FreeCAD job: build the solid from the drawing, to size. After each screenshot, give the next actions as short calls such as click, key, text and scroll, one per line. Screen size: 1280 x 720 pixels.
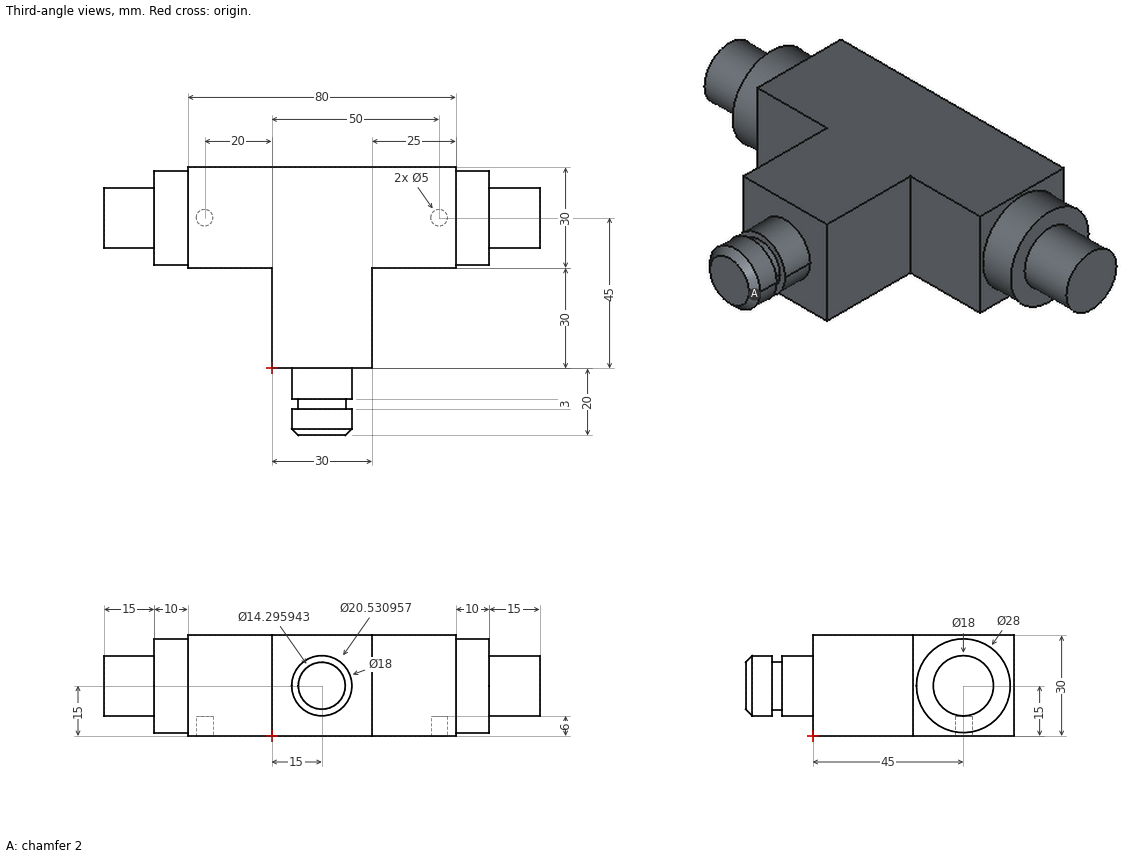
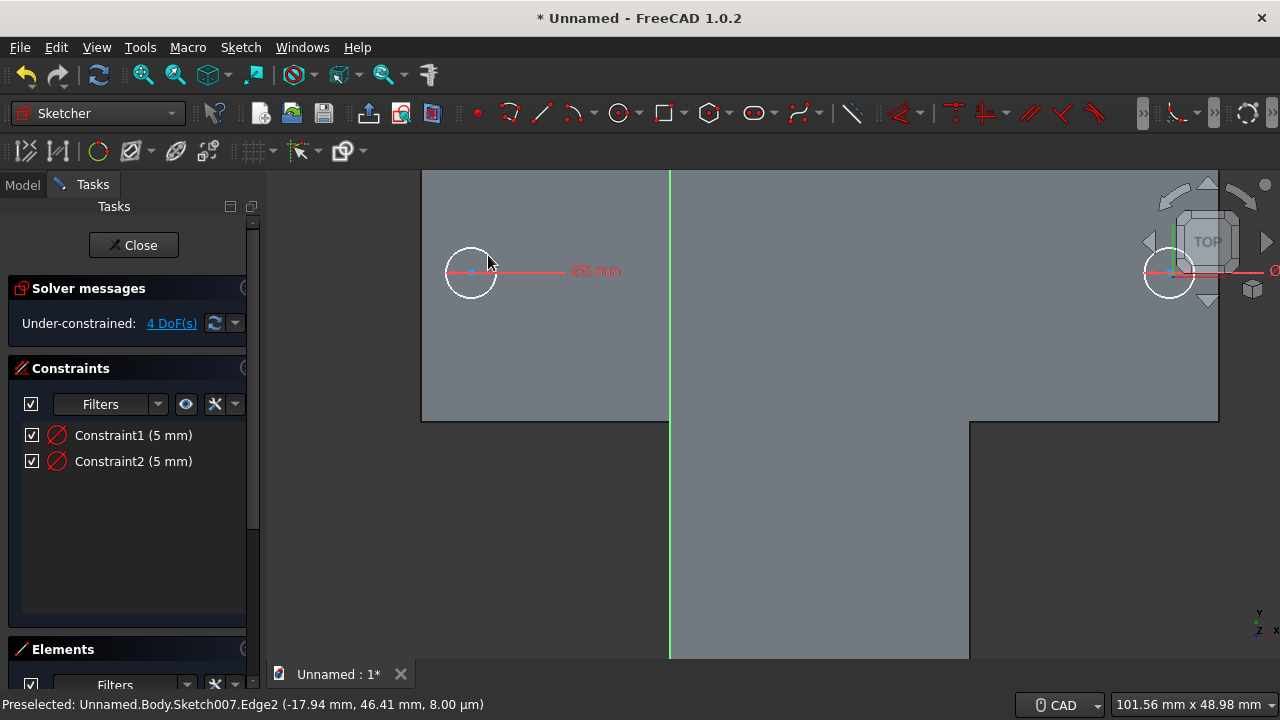
key(d)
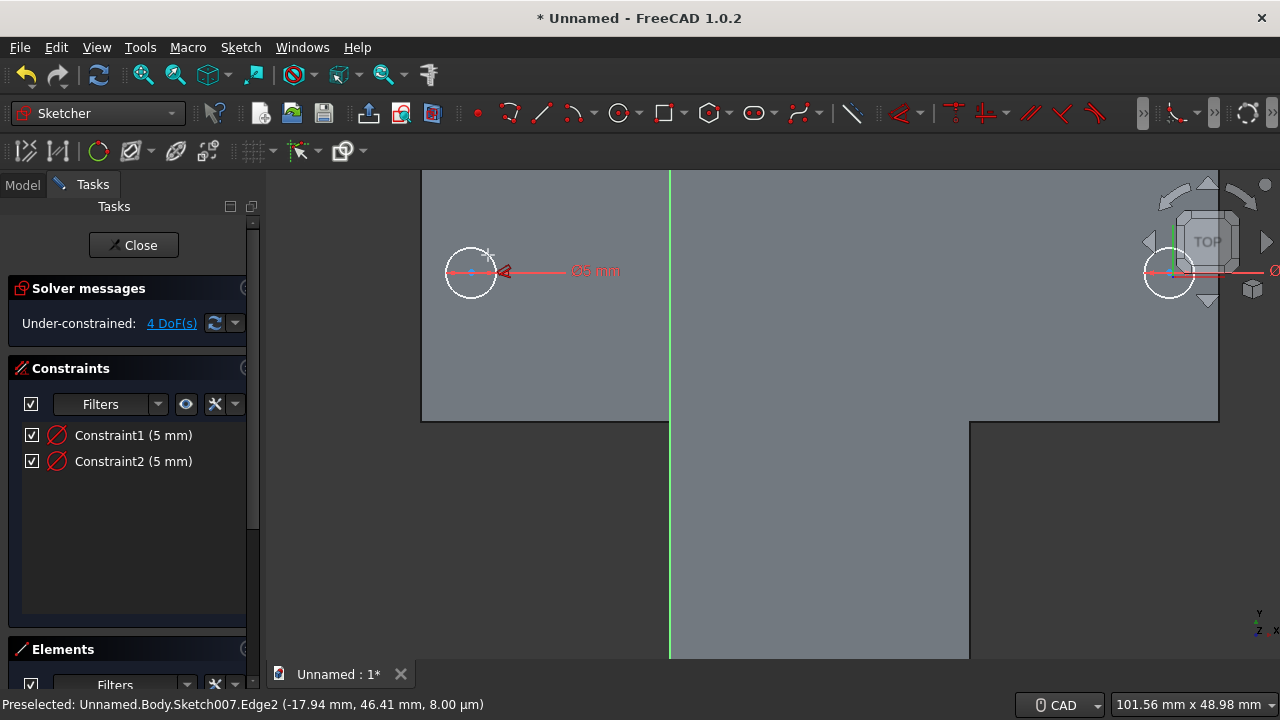
scroll(470, 272, down, 2)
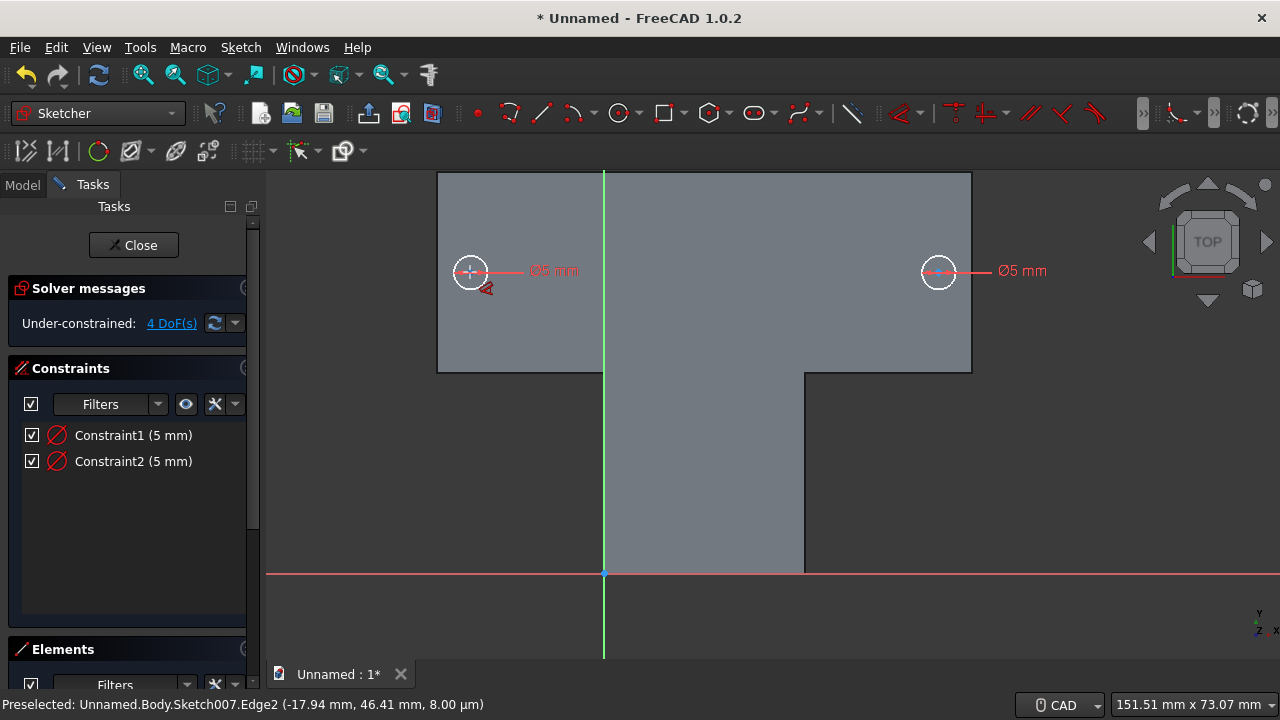
click(939, 273)
click(772, 608)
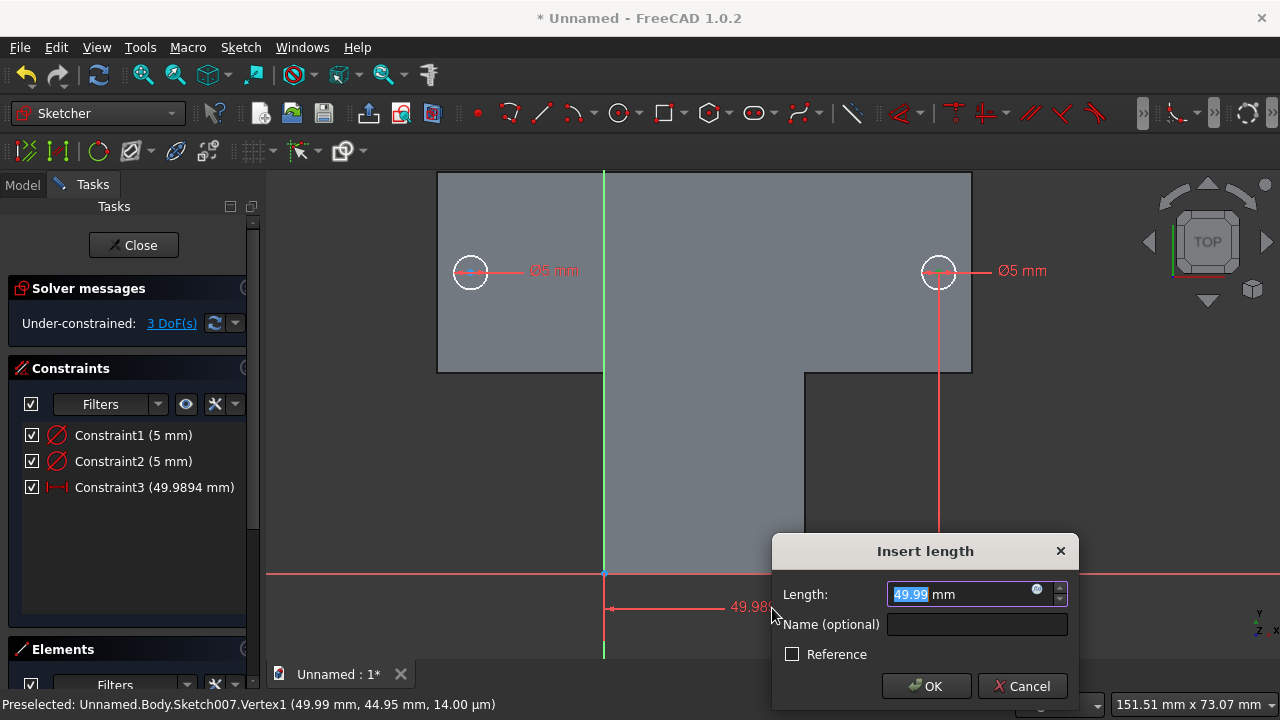
text(50)
key(Return)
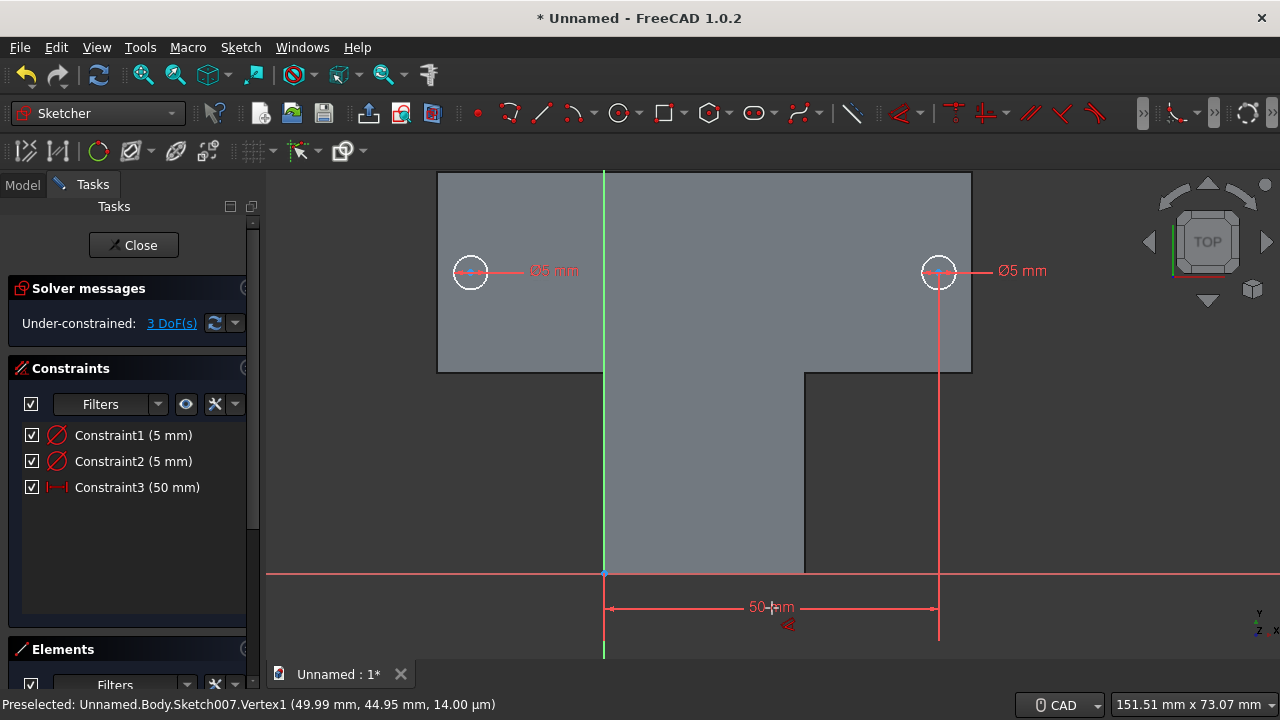
click(939, 273)
click(973, 423)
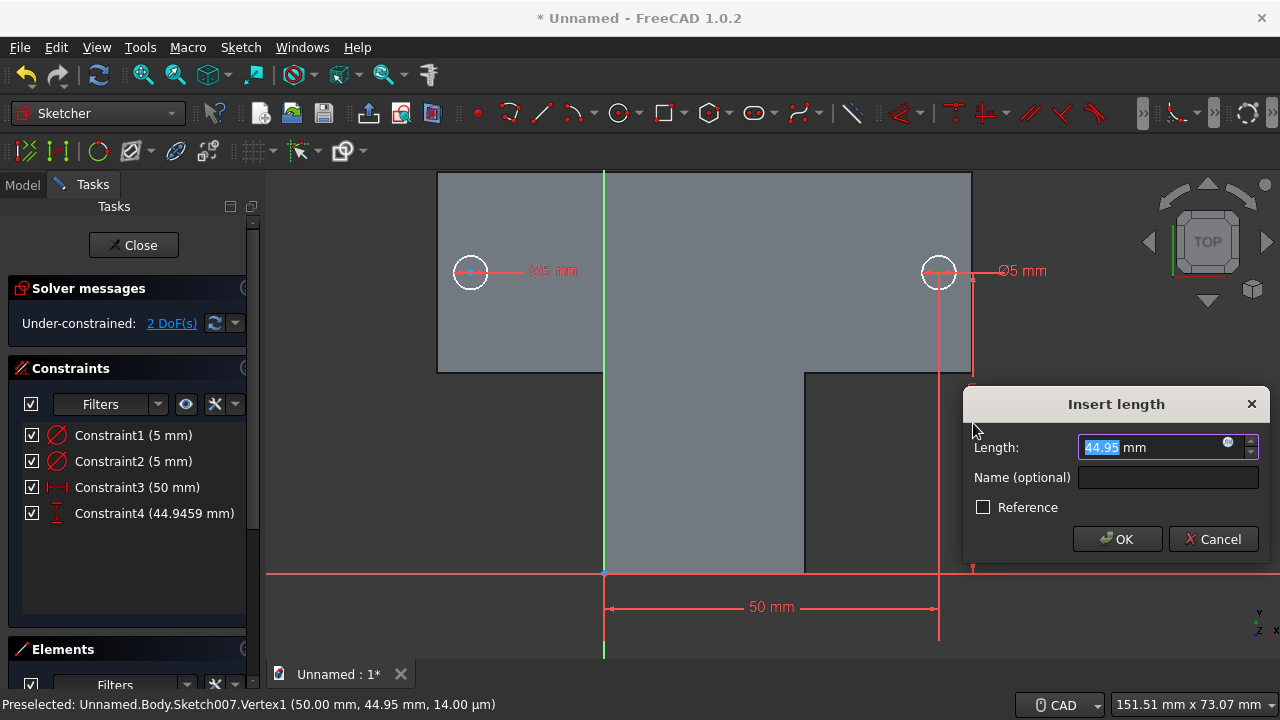
text(45)
key(Return)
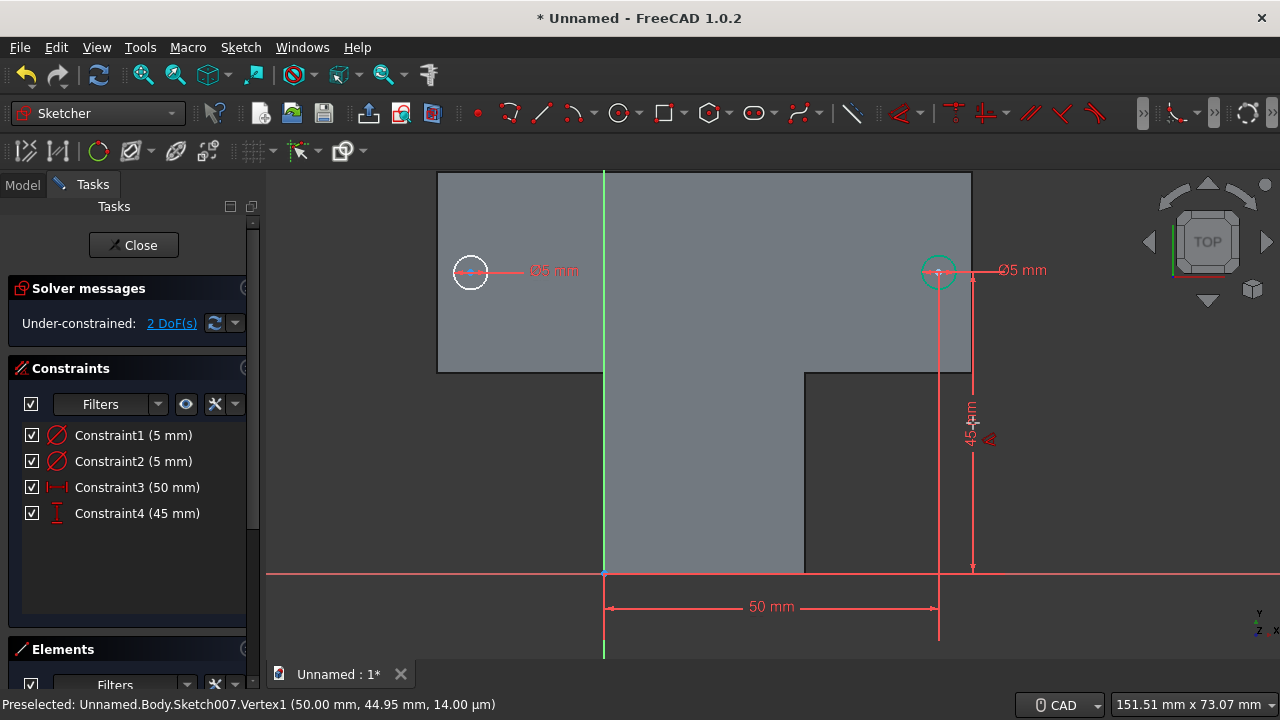
click(471, 273)
click(538, 608)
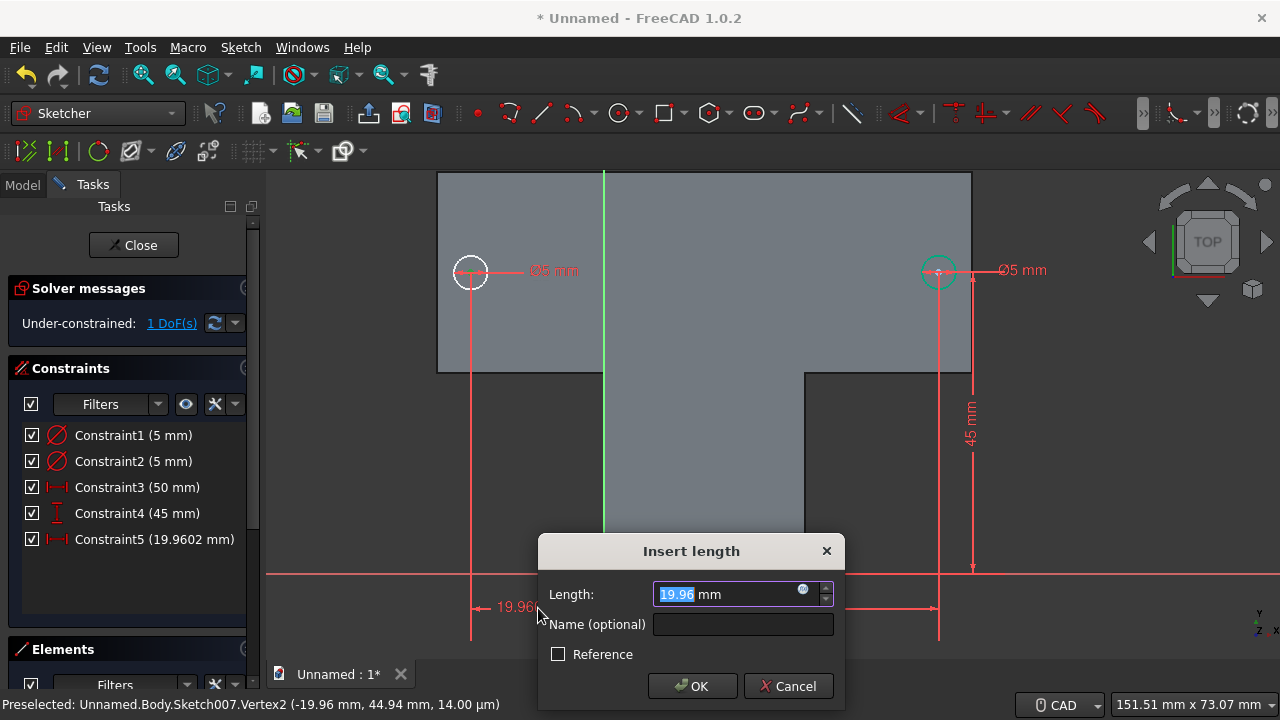
text(20)
key(Return)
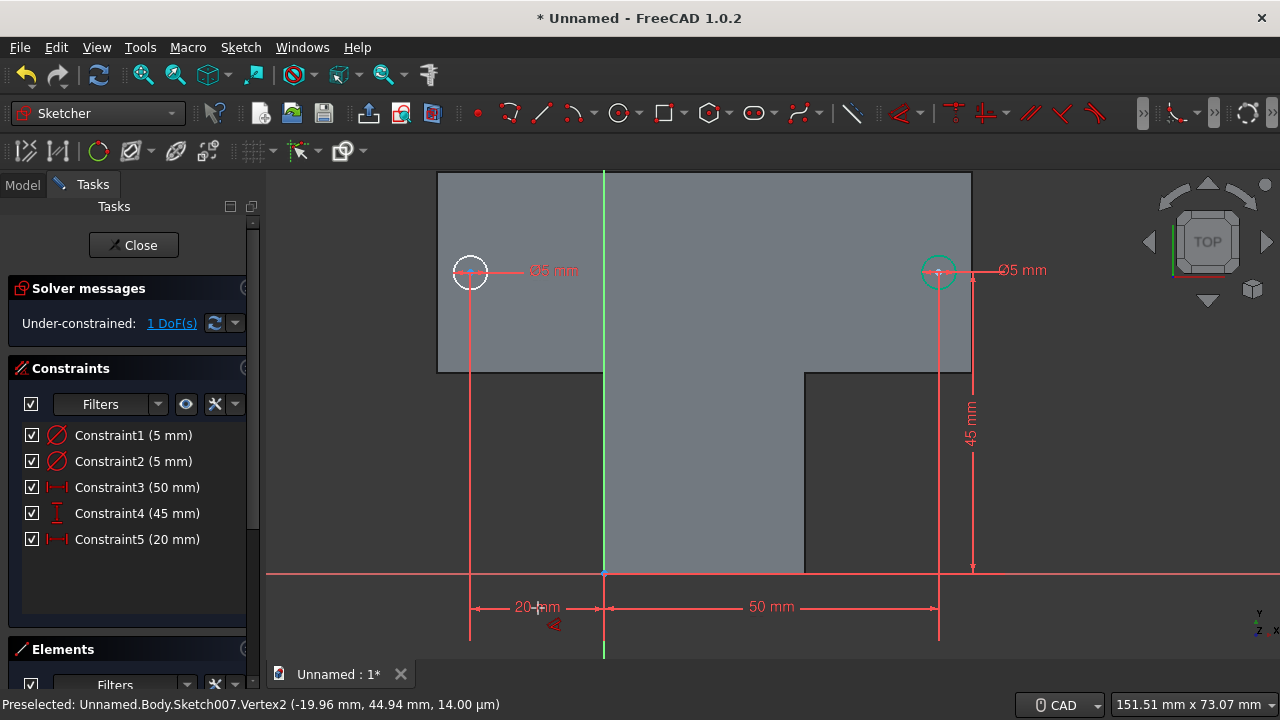
click(470, 273)
click(436, 423)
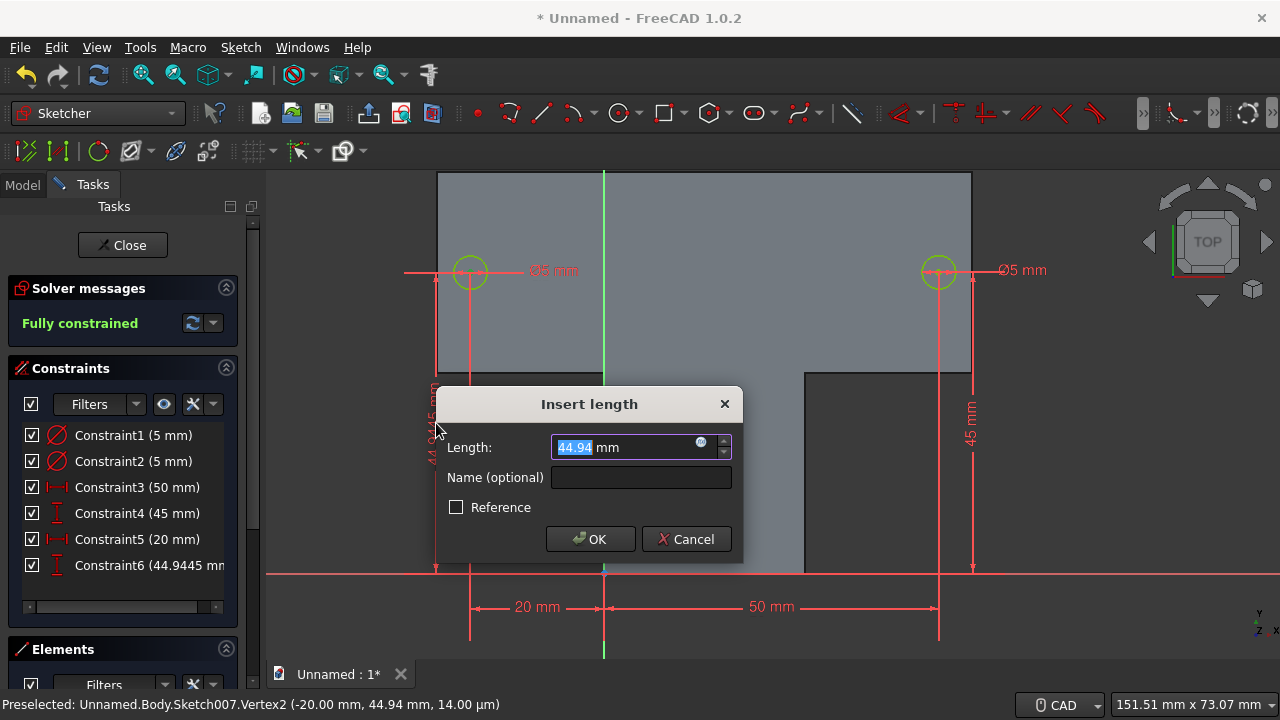
text(45)
key(Return)
key(Escape)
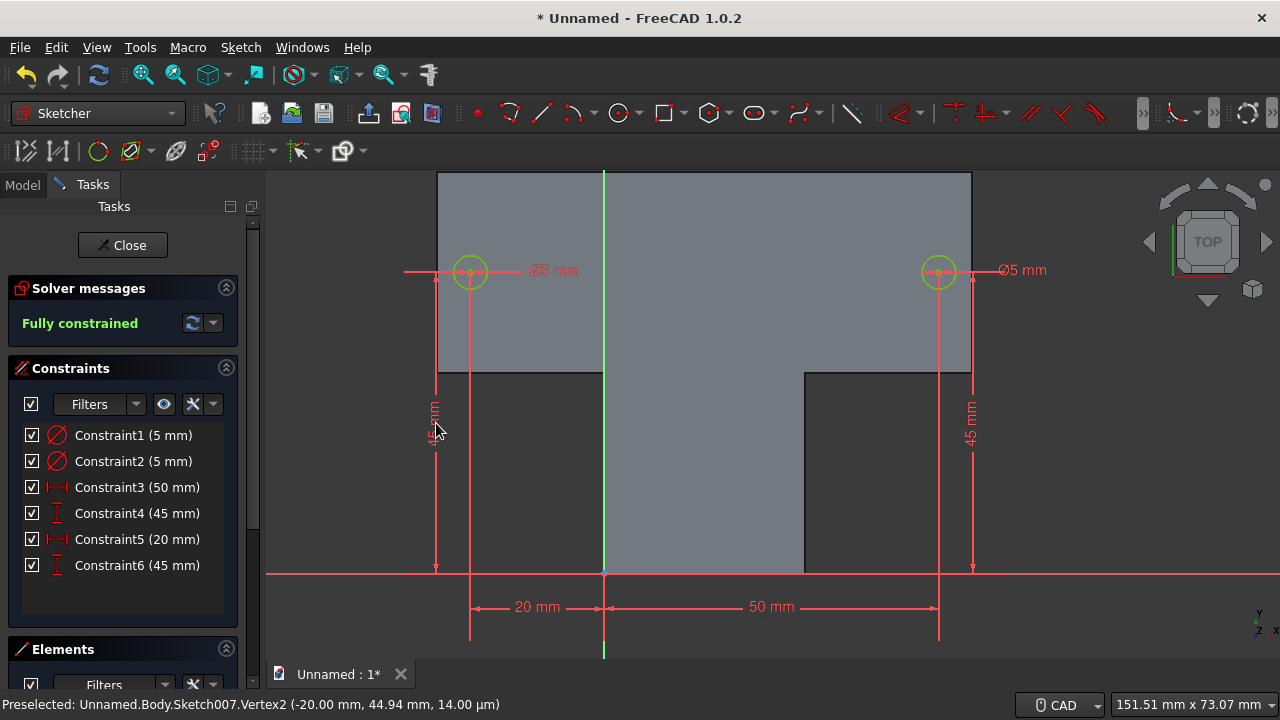
click(123, 245)